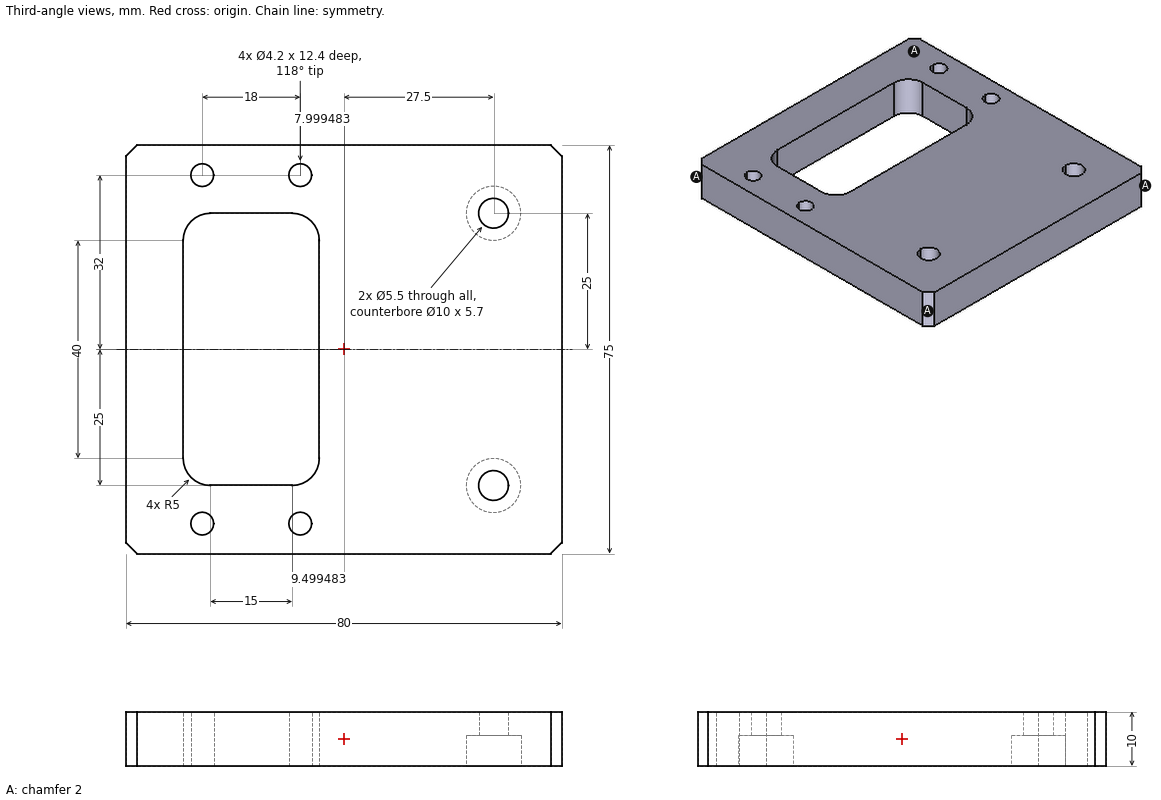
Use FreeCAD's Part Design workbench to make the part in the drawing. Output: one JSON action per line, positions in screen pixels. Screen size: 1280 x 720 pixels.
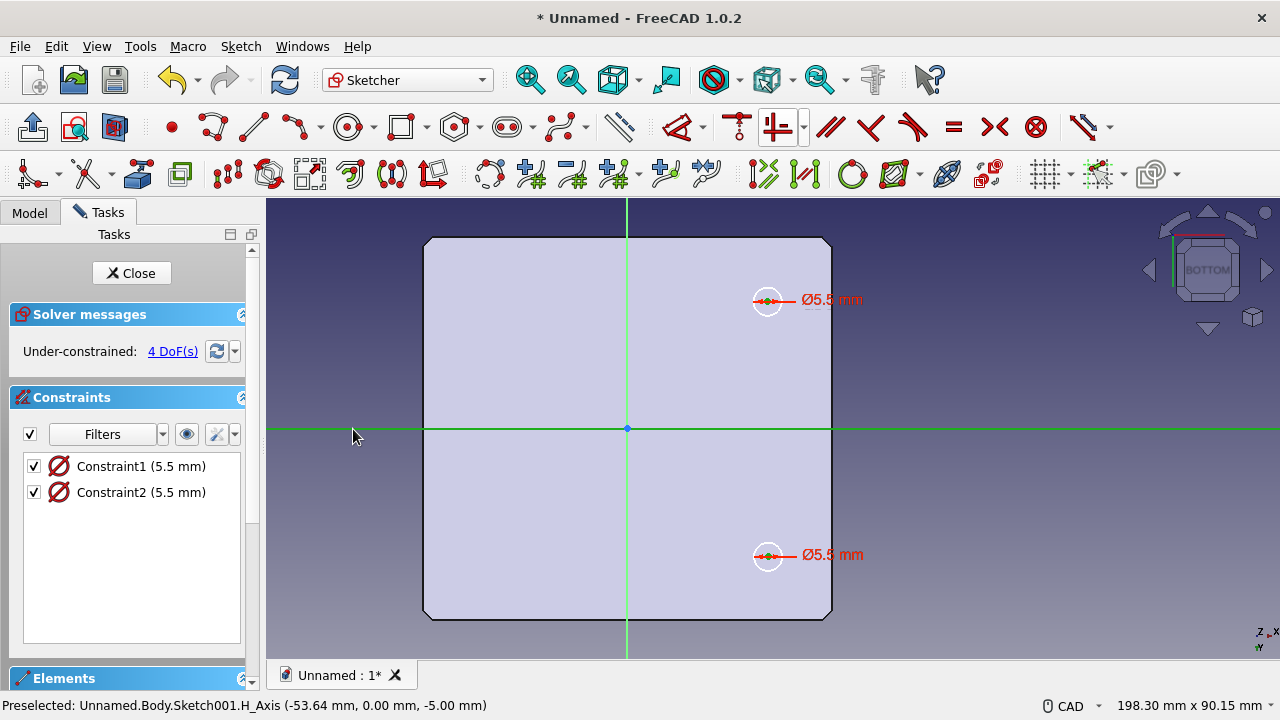
{"action": "key", "text": "s"}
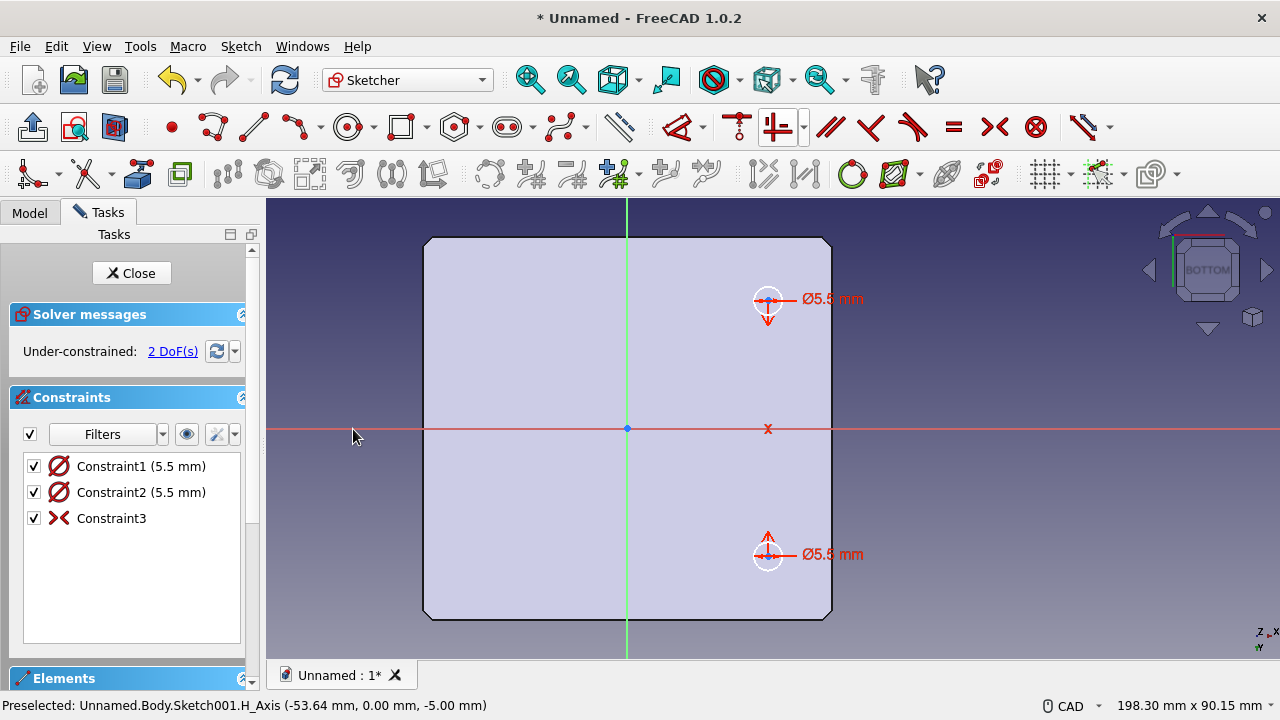
{"action": "key", "text": "d"}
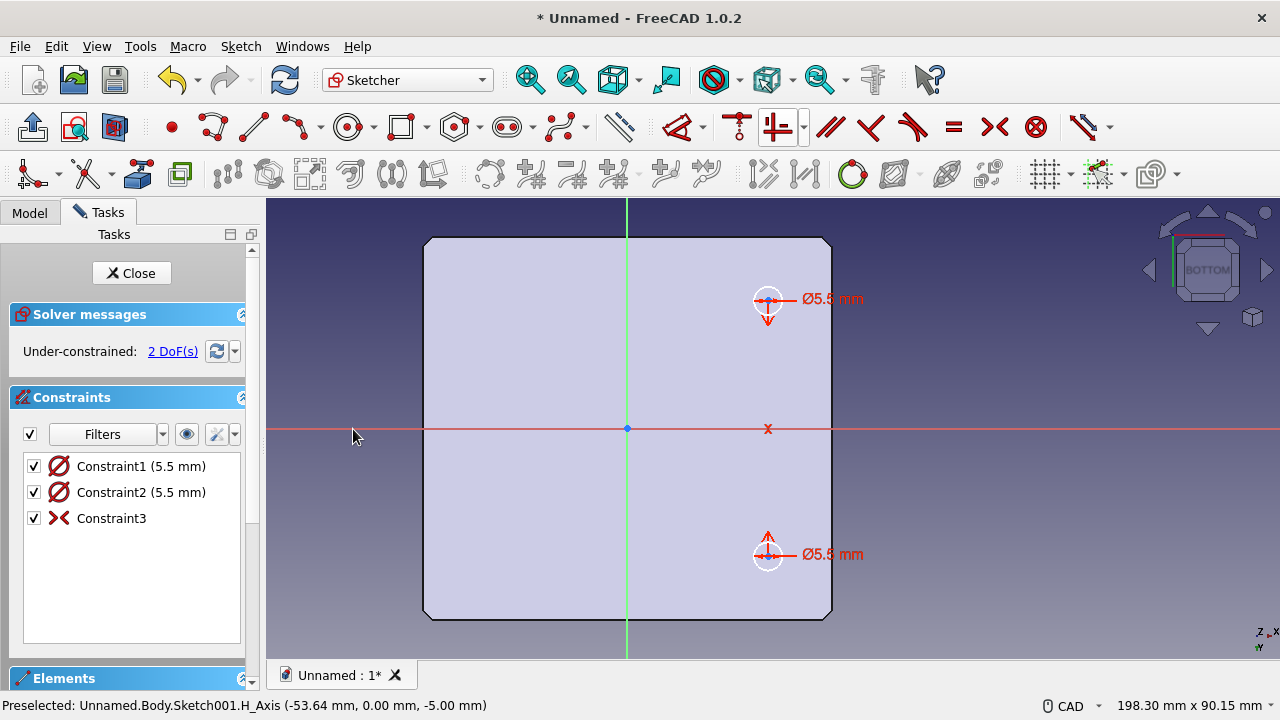
{"action": "left_click", "coordinate": [768, 556]}
{"action": "left_click", "coordinate": [593, 493]}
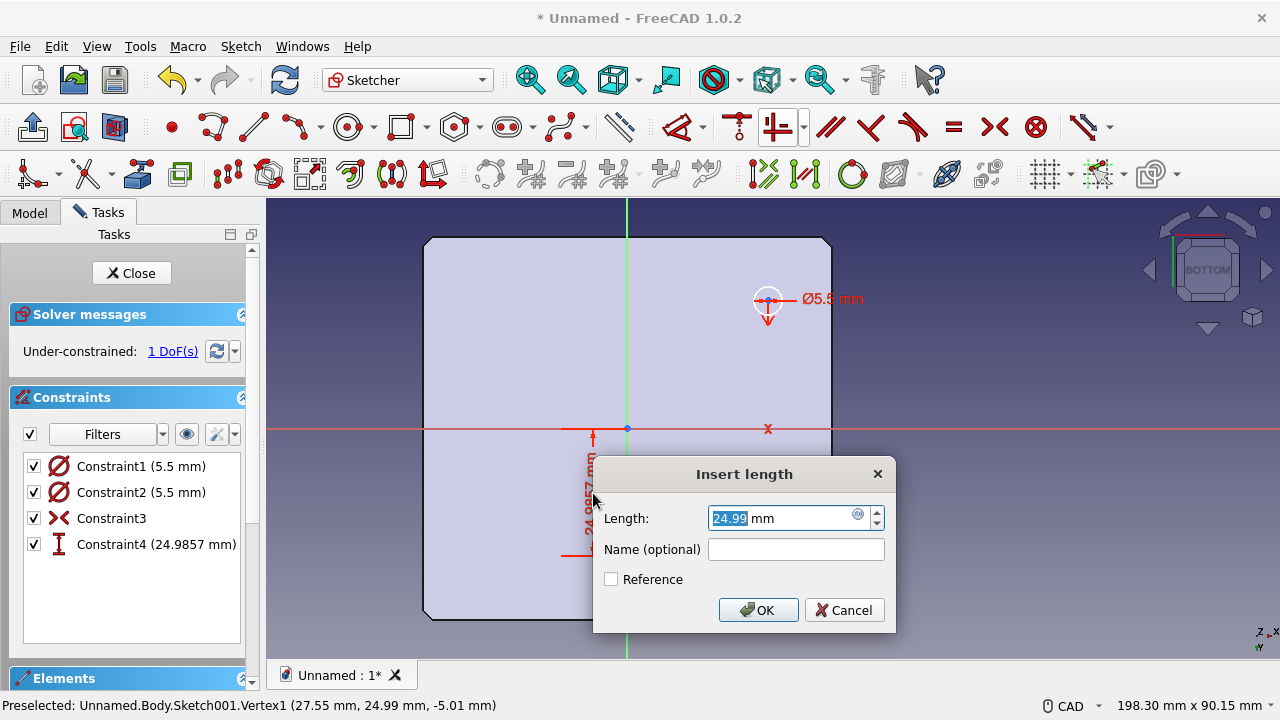
{"action": "type", "text": "25"}
{"action": "key", "text": "Return"}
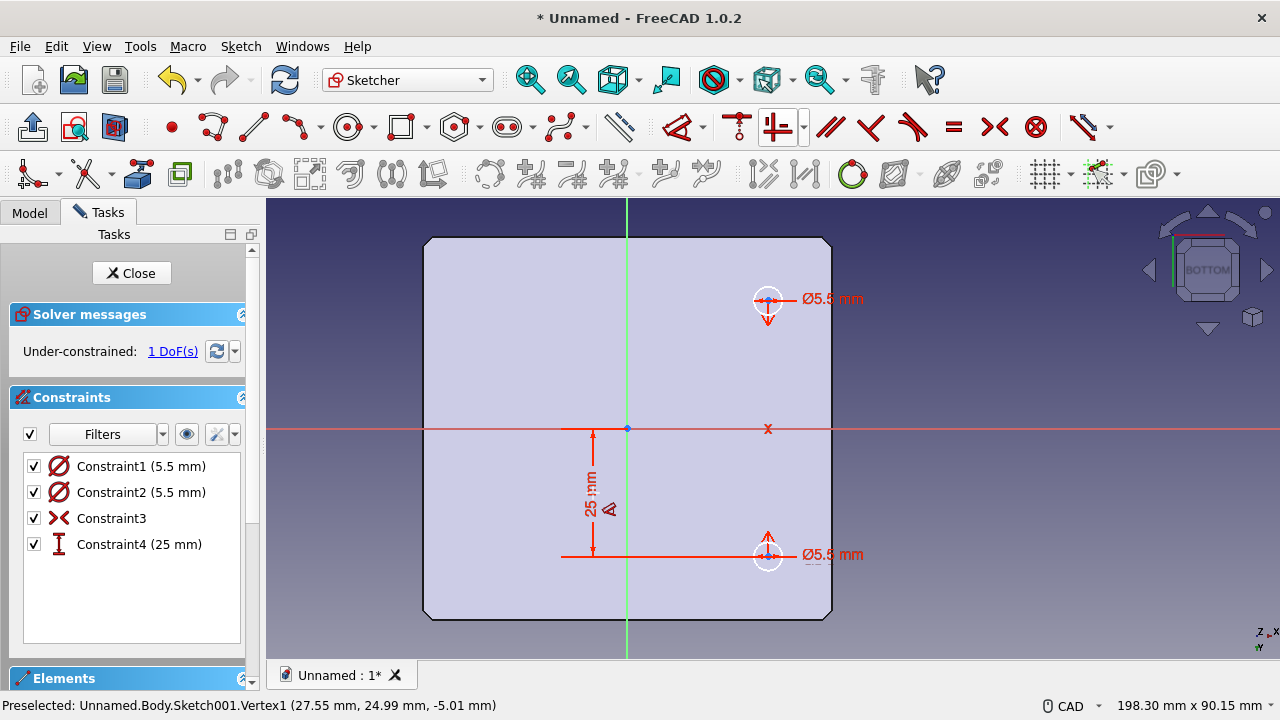
{"action": "left_click", "coordinate": [768, 557]}
{"action": "left_click", "coordinate": [698, 591]}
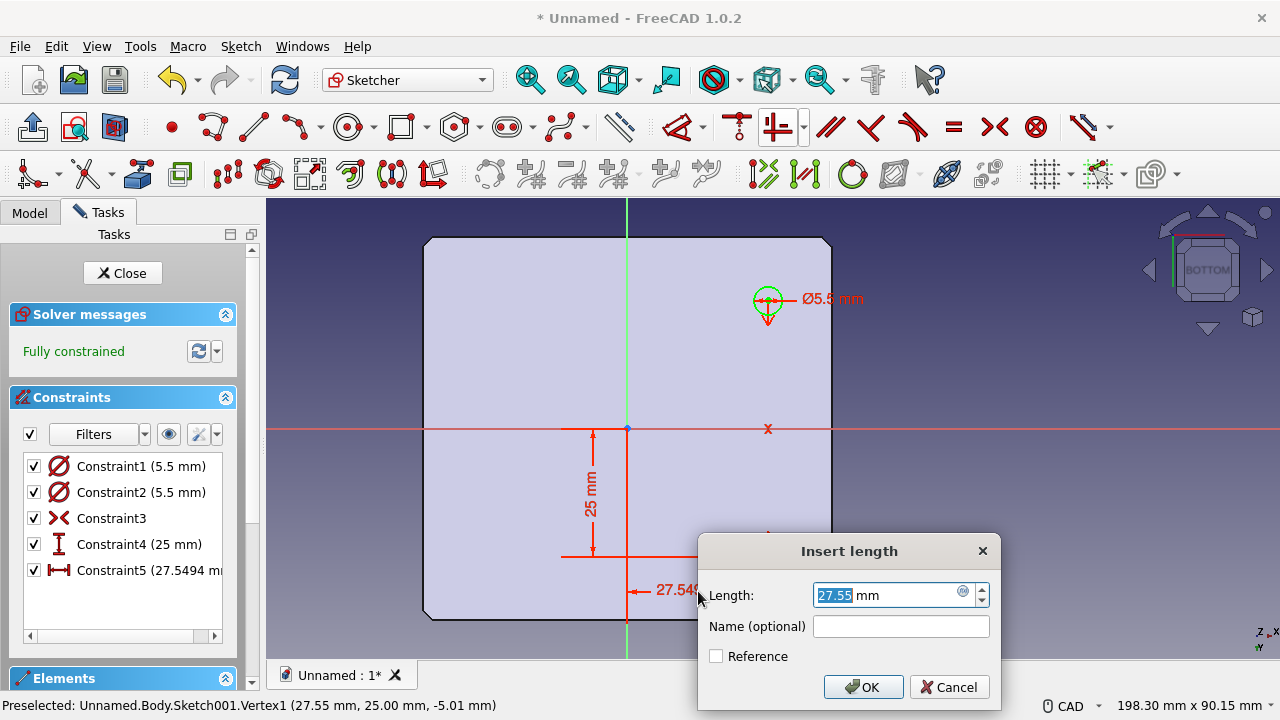
{"action": "type", "text": "27.5"}
{"action": "key", "text": "Return"}
{"action": "key", "text": "Escape"}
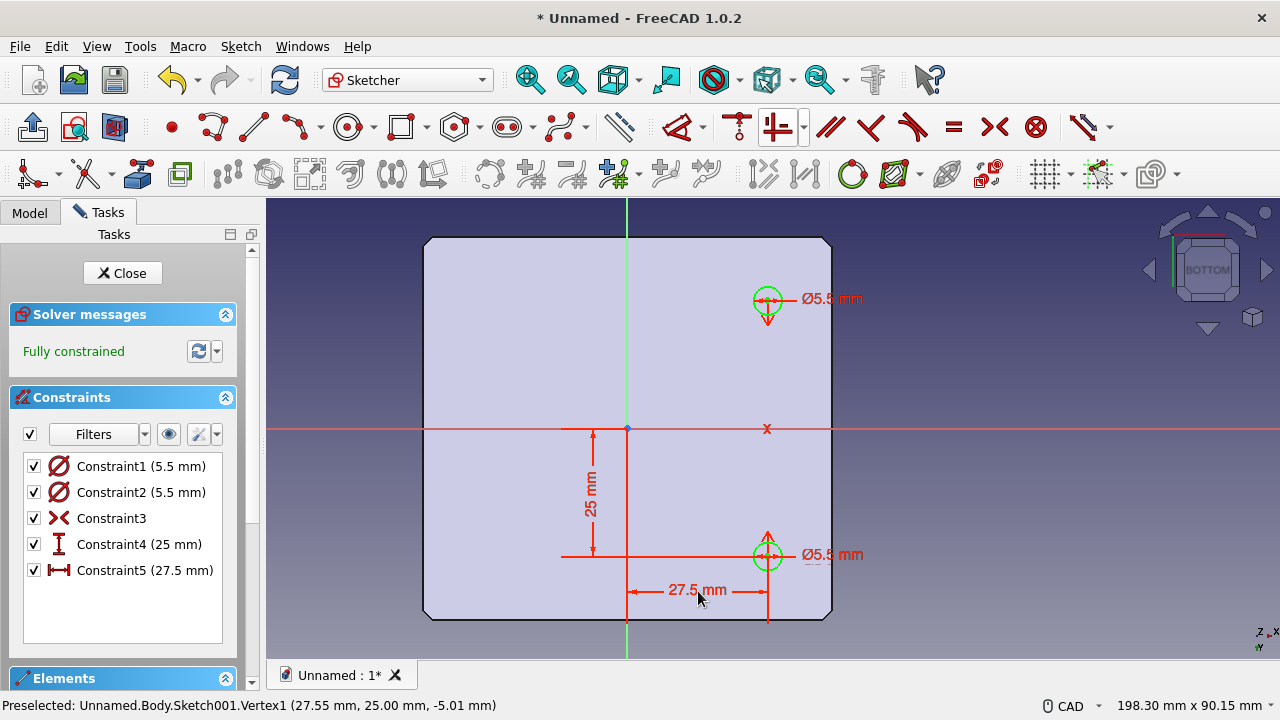
{"action": "left_click", "coordinate": [123, 273]}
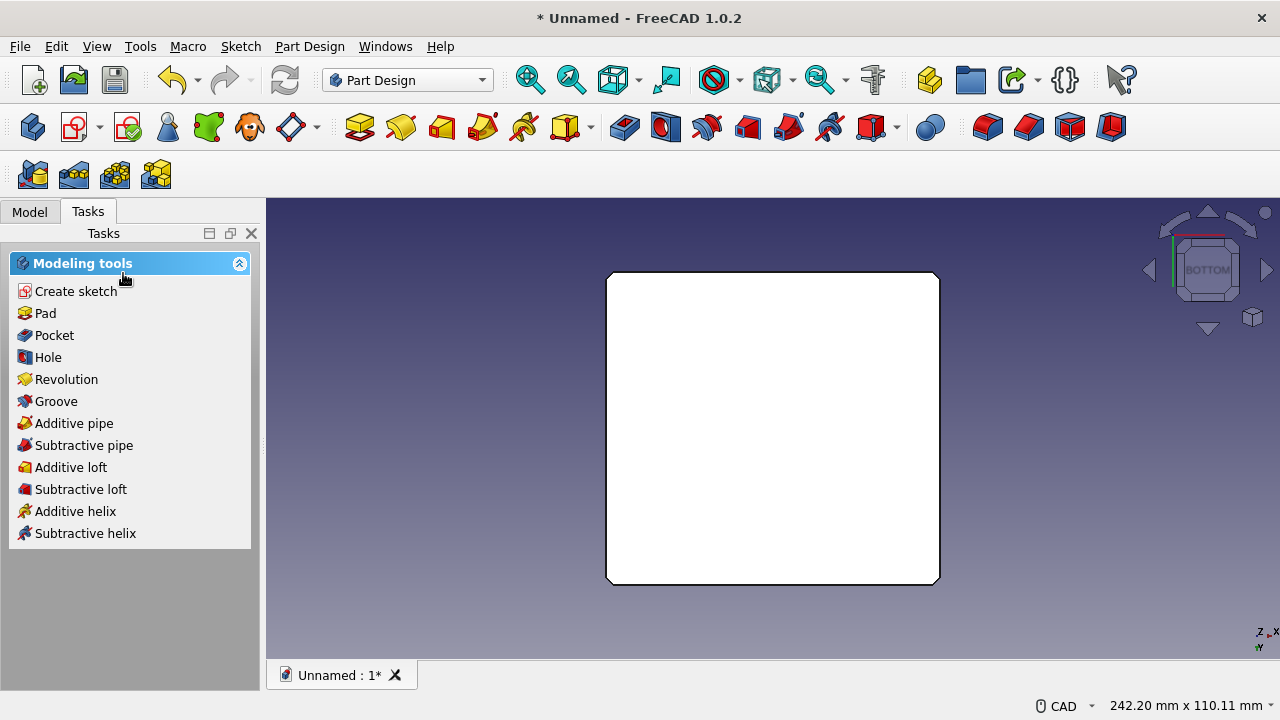
{"action": "left_click", "coordinate": [666, 128]}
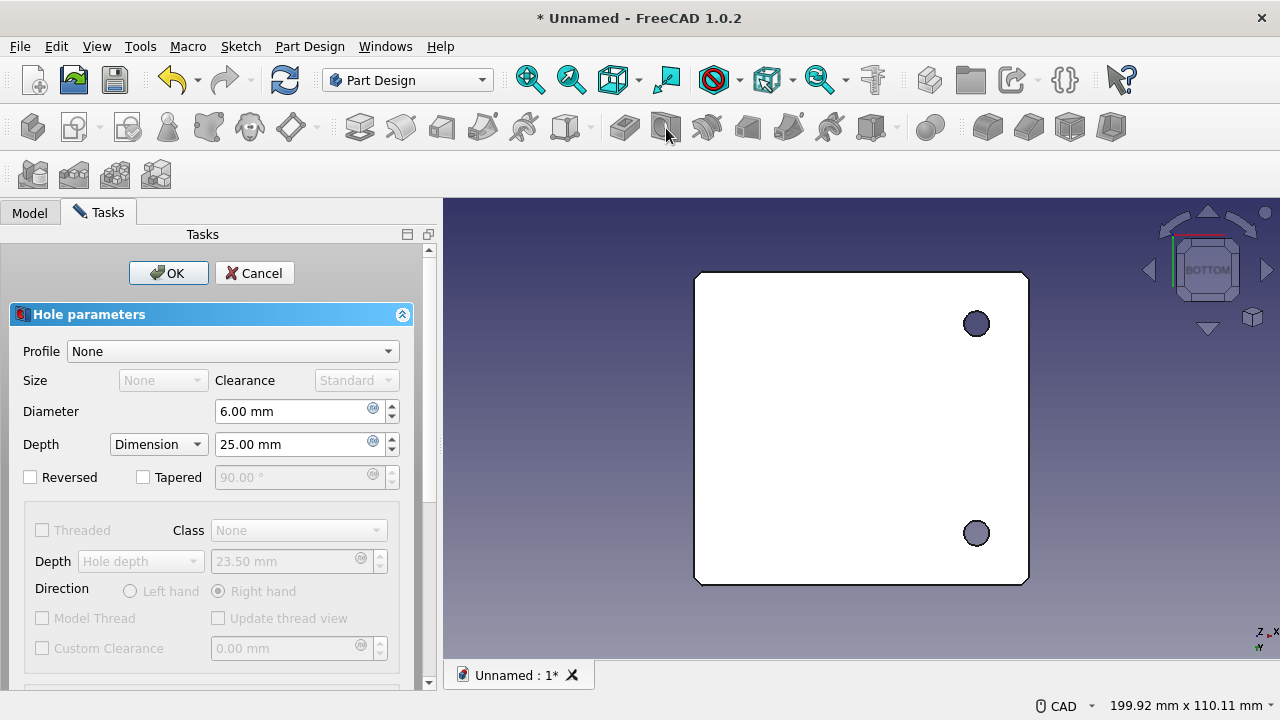
{"action": "triple_click", "coordinate": [300, 412]}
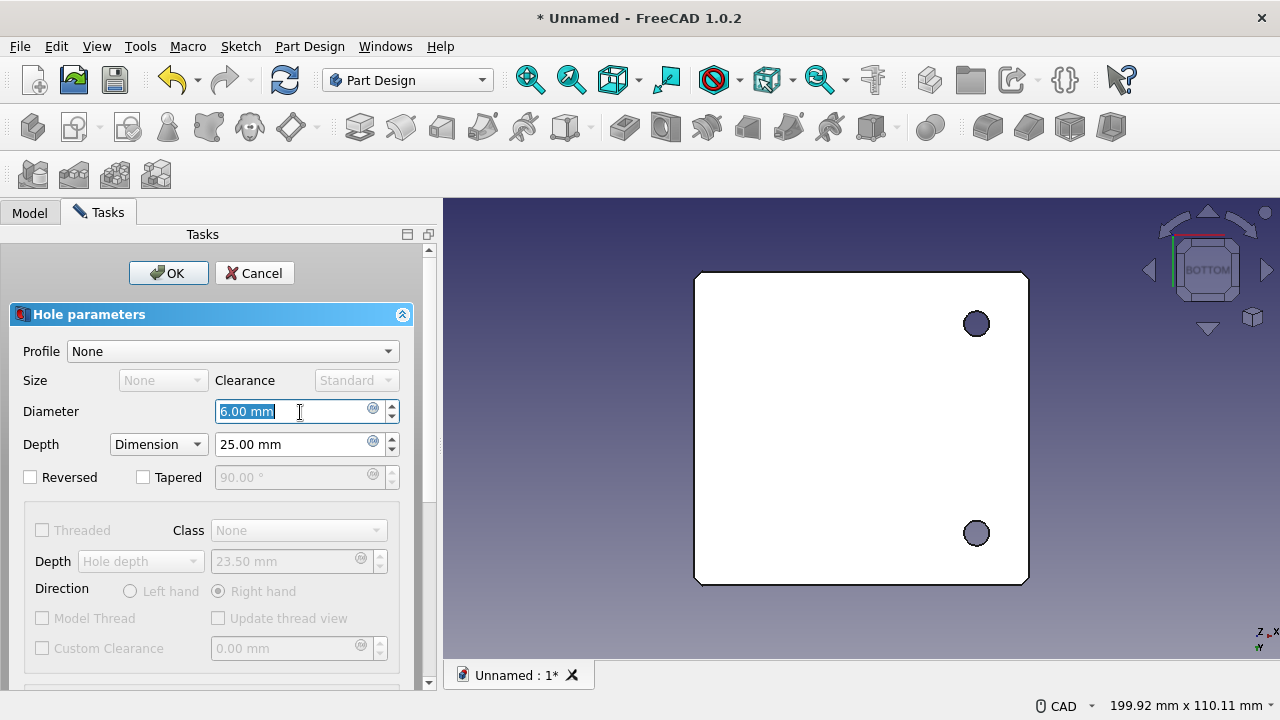
{"action": "type", "text": "5.5"}
{"action": "key", "text": "Tab"}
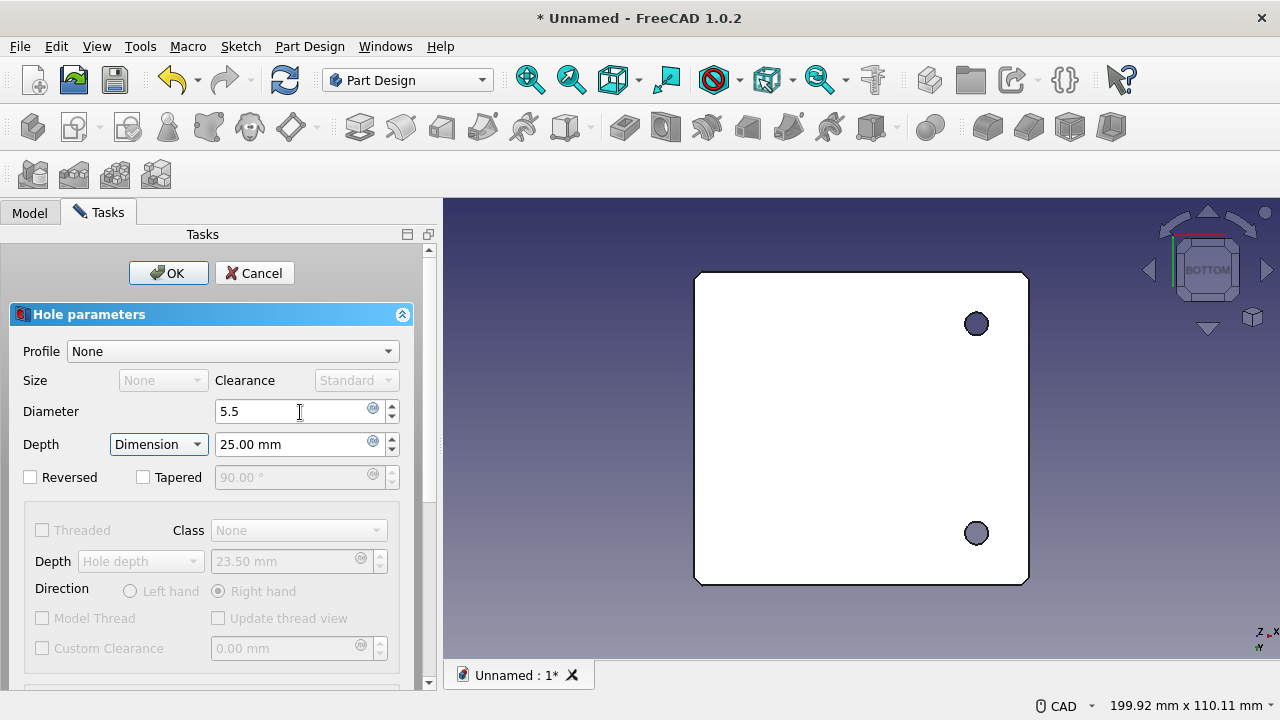
{"action": "left_click", "coordinate": [160, 444]}